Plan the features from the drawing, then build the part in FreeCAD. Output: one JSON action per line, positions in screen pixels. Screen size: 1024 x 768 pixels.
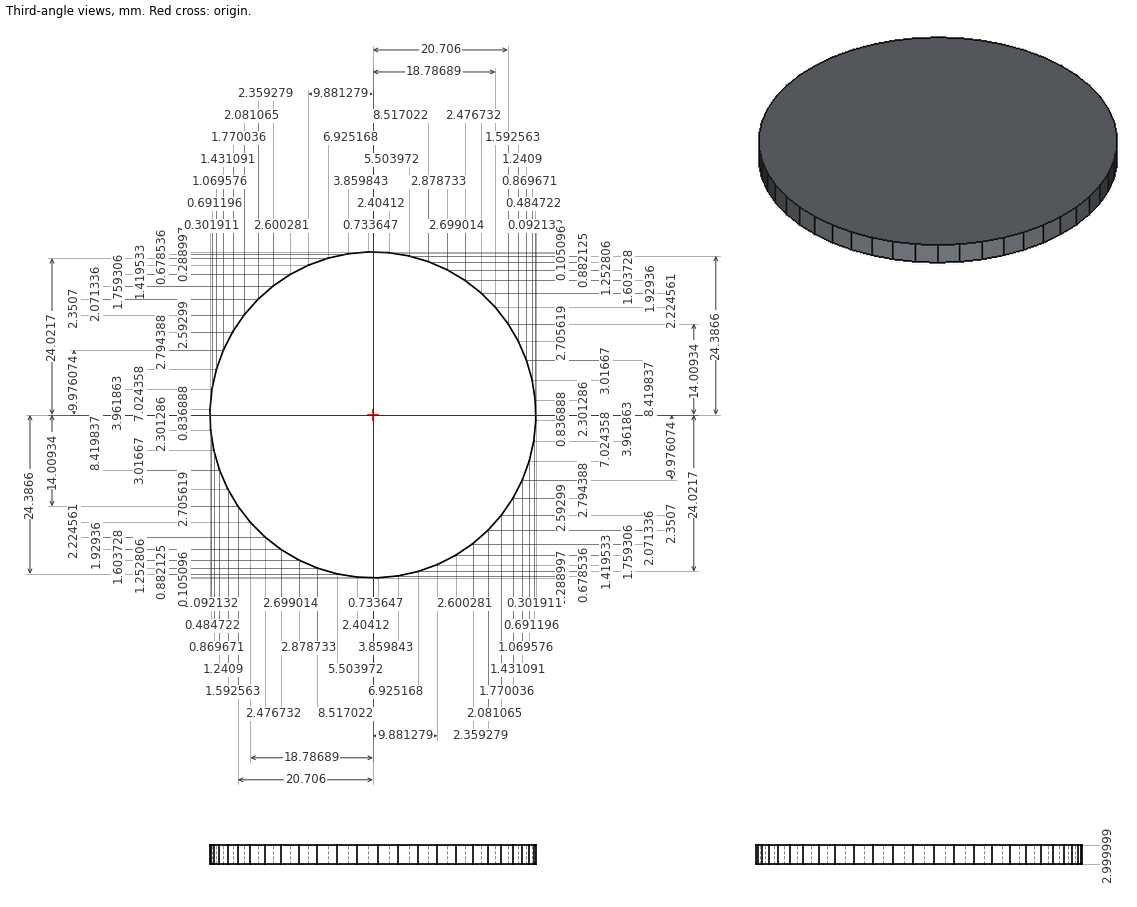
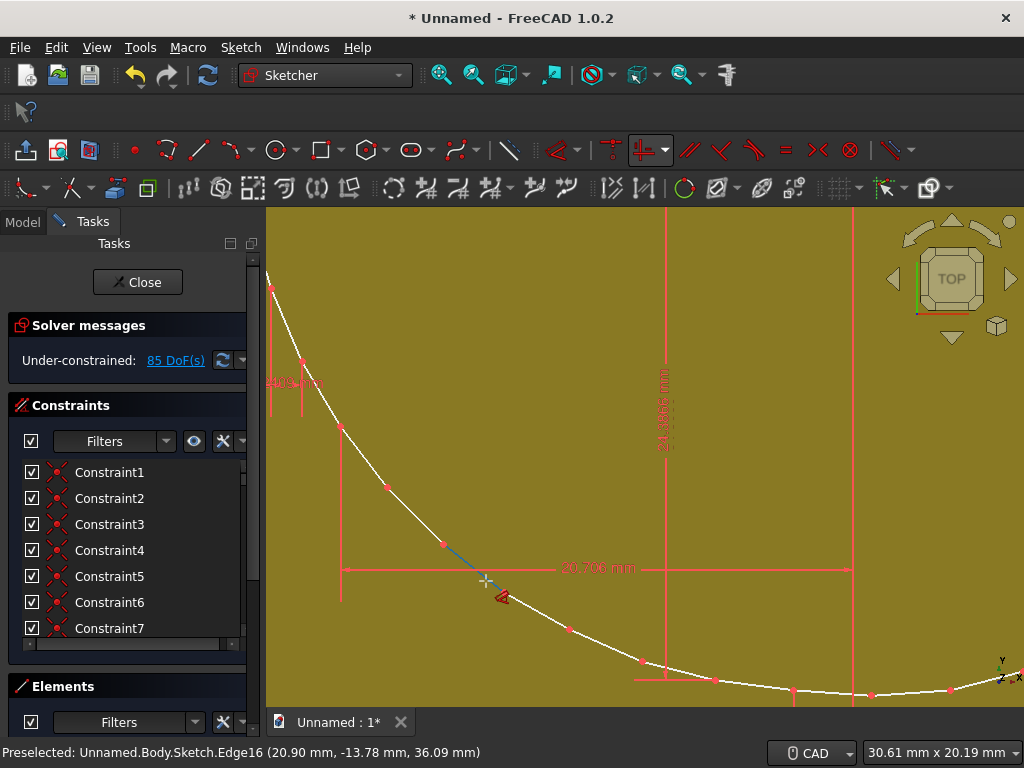
{"action": "left_click", "coordinate": [487, 578]}
{"action": "left_click", "coordinate": [410, 569]}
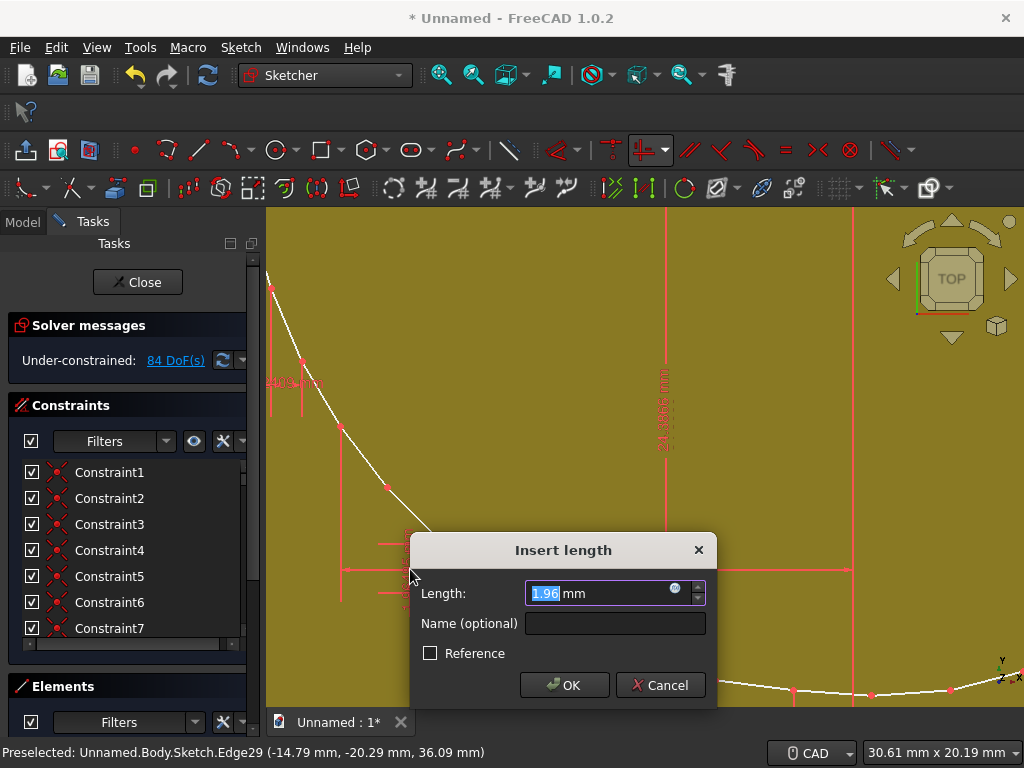
{"action": "type", "text": "1.92936"}
{"action": "key", "text": "Return"}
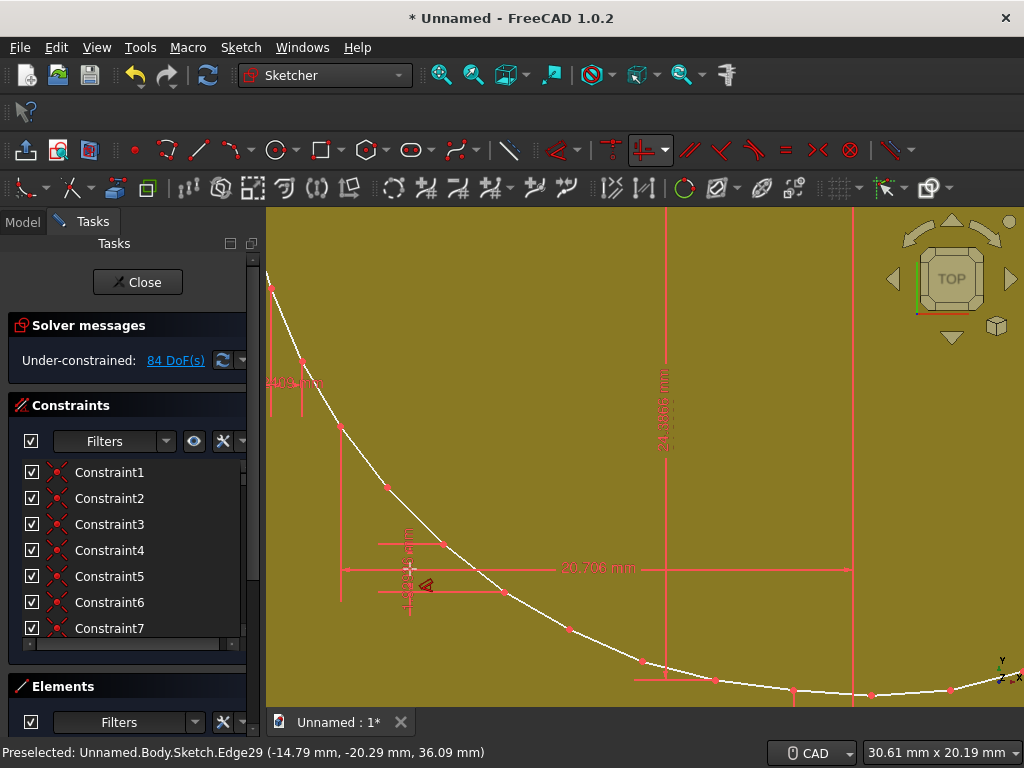
{"action": "scroll", "coordinate": [486, 582], "scroll_direction": "down", "scroll_amount": 7}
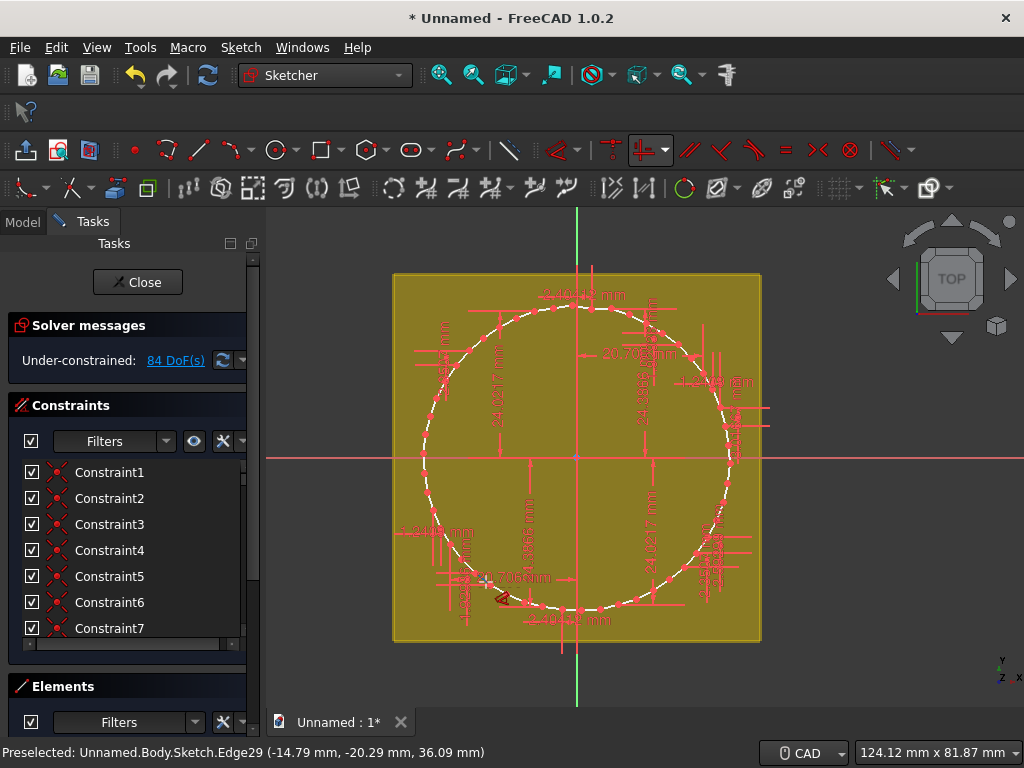
{"action": "scroll", "coordinate": [432, 505], "scroll_direction": "up", "scroll_amount": 5}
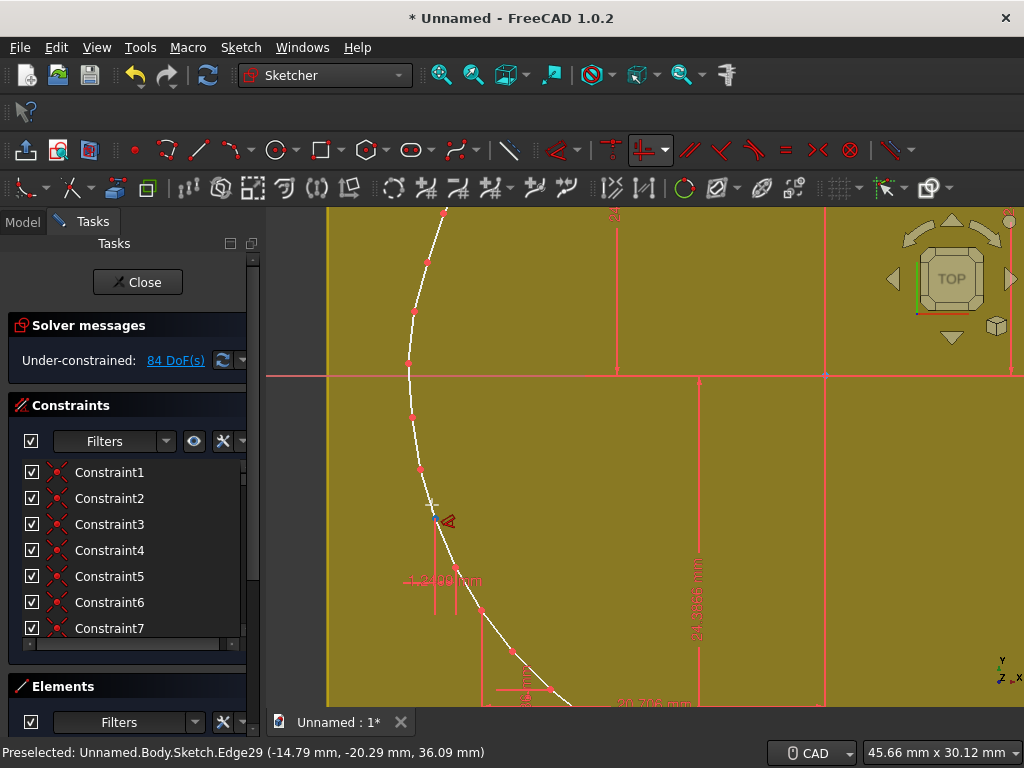
{"action": "left_click", "coordinate": [431, 504]}
{"action": "left_click", "coordinate": [386, 494]}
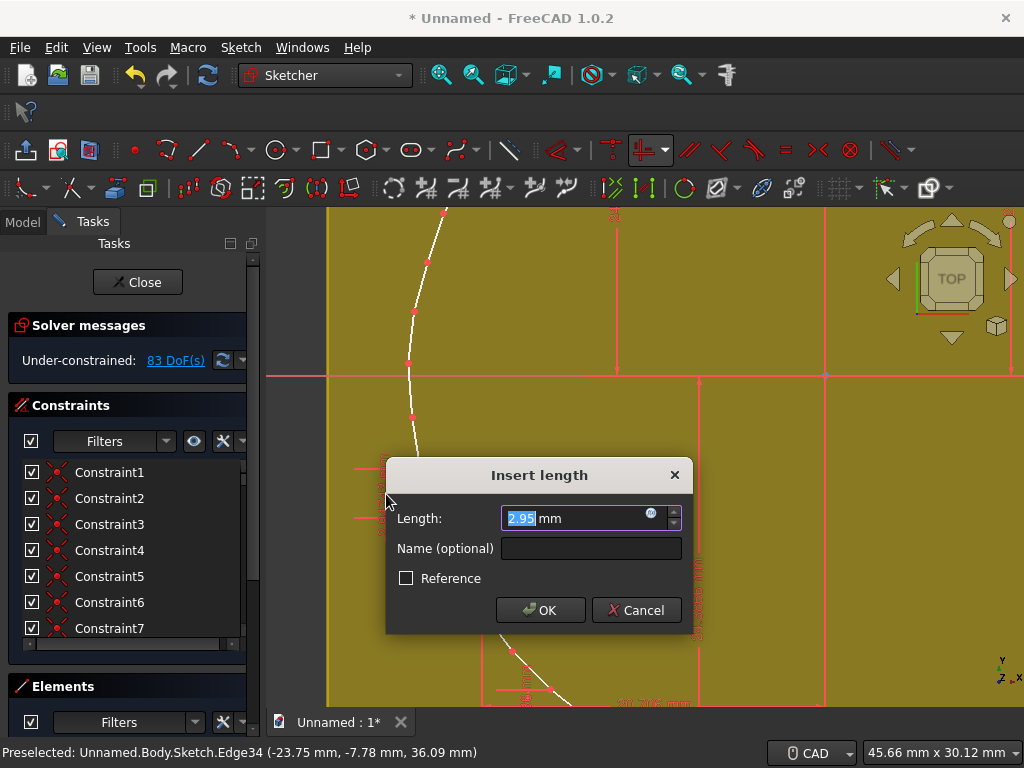
{"action": "type", "text": "3.01667"}
{"action": "key", "text": "Return"}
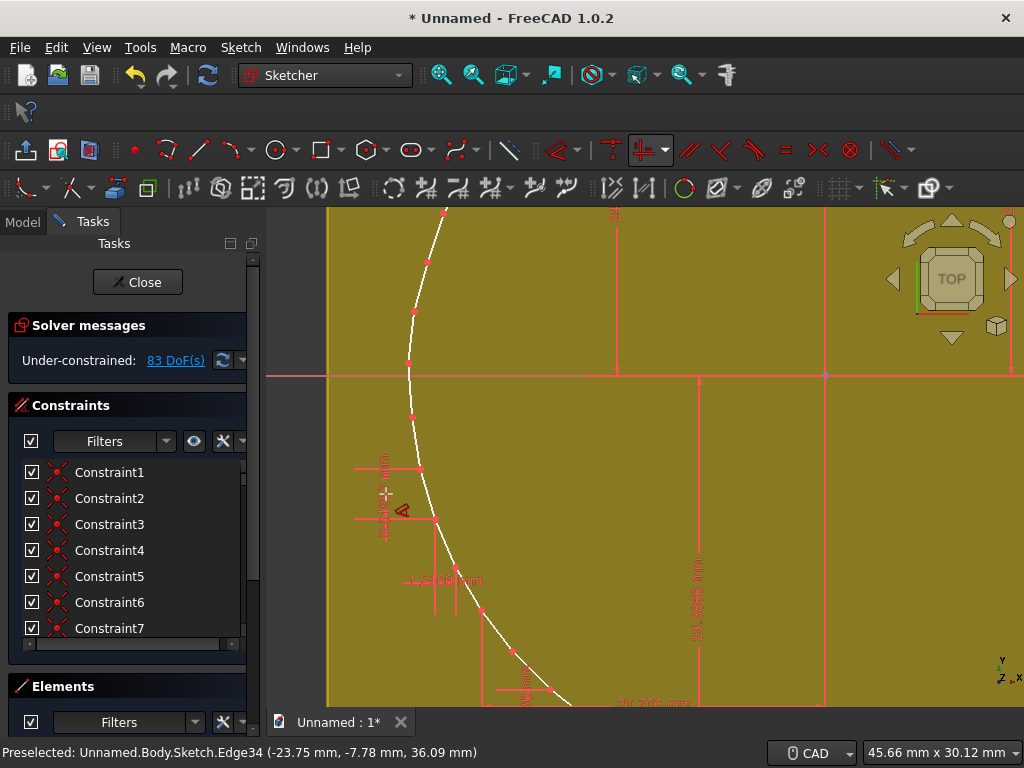
{"action": "scroll", "coordinate": [432, 504], "scroll_direction": "down", "scroll_amount": 5}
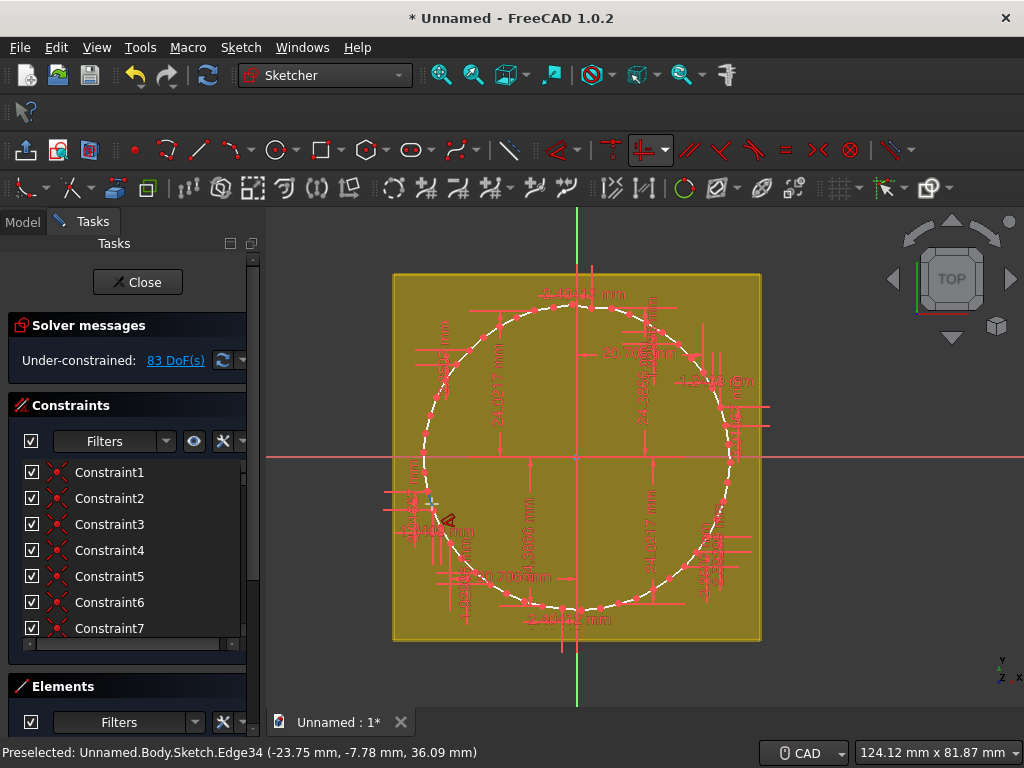
{"action": "scroll", "coordinate": [449, 376], "scroll_direction": "up", "scroll_amount": 5}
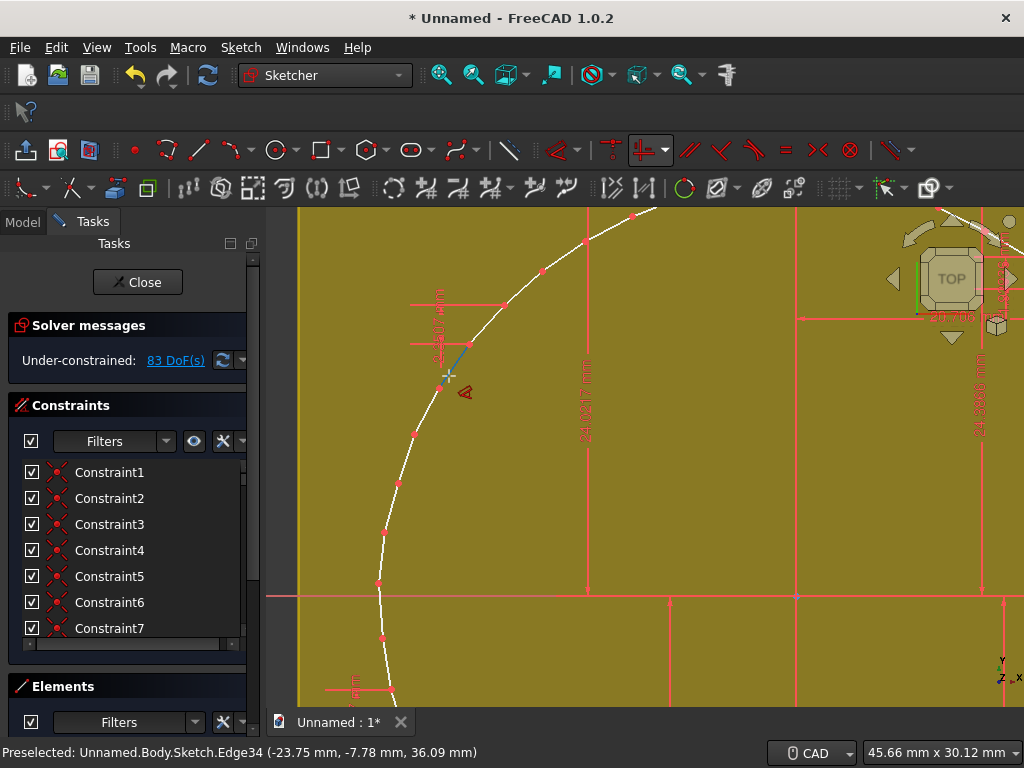
{"action": "left_click", "coordinate": [448, 375]}
{"action": "left_click", "coordinate": [405, 366]}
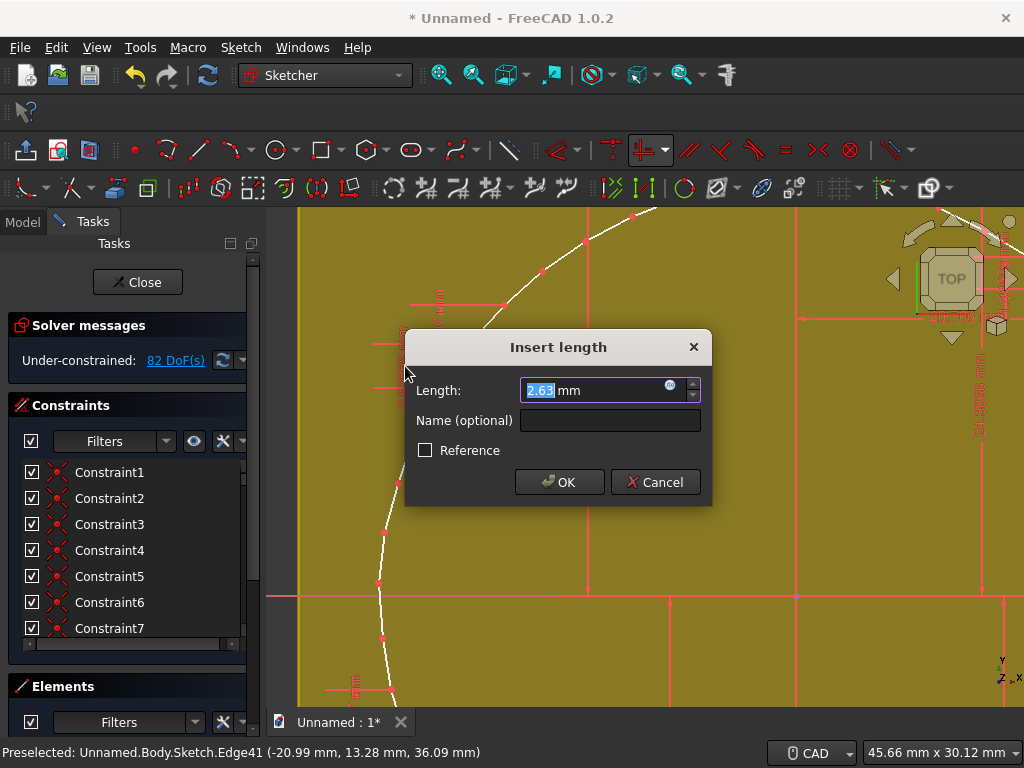
{"action": "type", "text": "2.59299"}
{"action": "key", "text": "Return"}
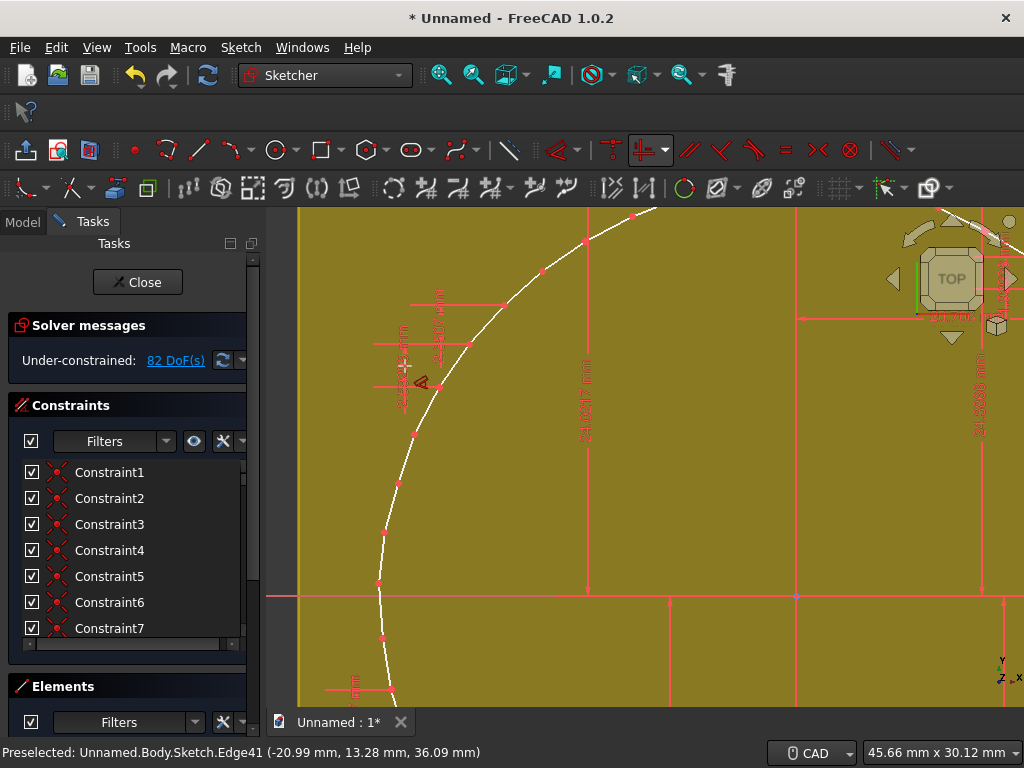
{"action": "scroll", "coordinate": [449, 376], "scroll_direction": "down", "scroll_amount": 5}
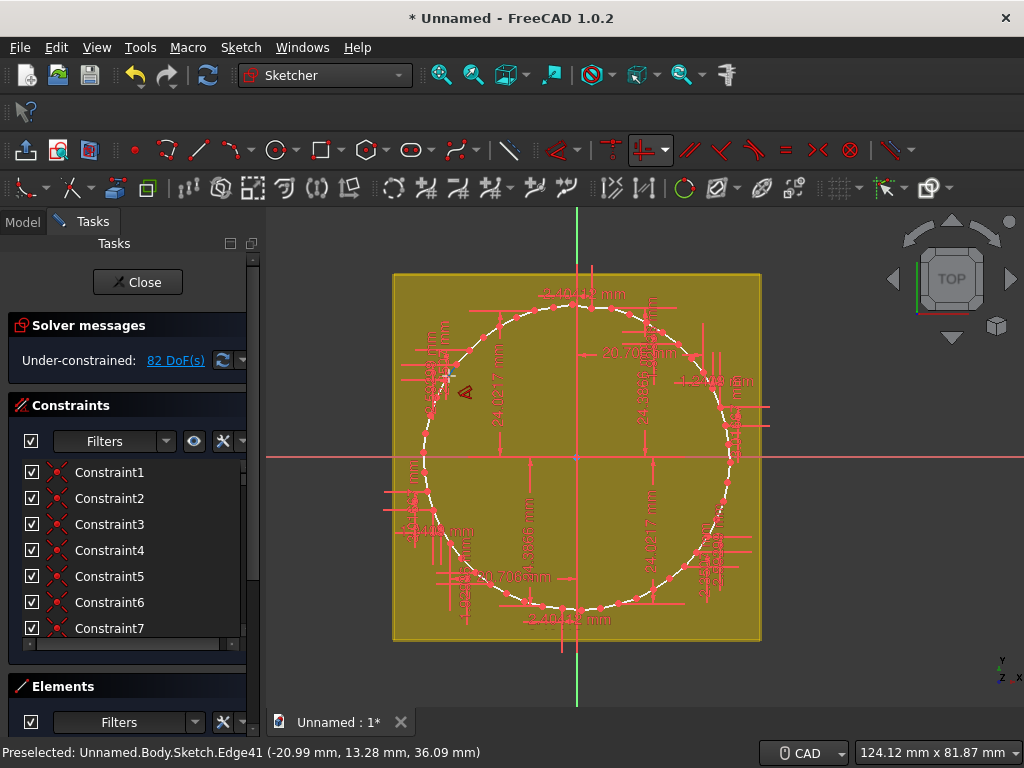
{"action": "left_click", "coordinate": [611, 308]}
{"action": "left_click", "coordinate": [594, 274]}